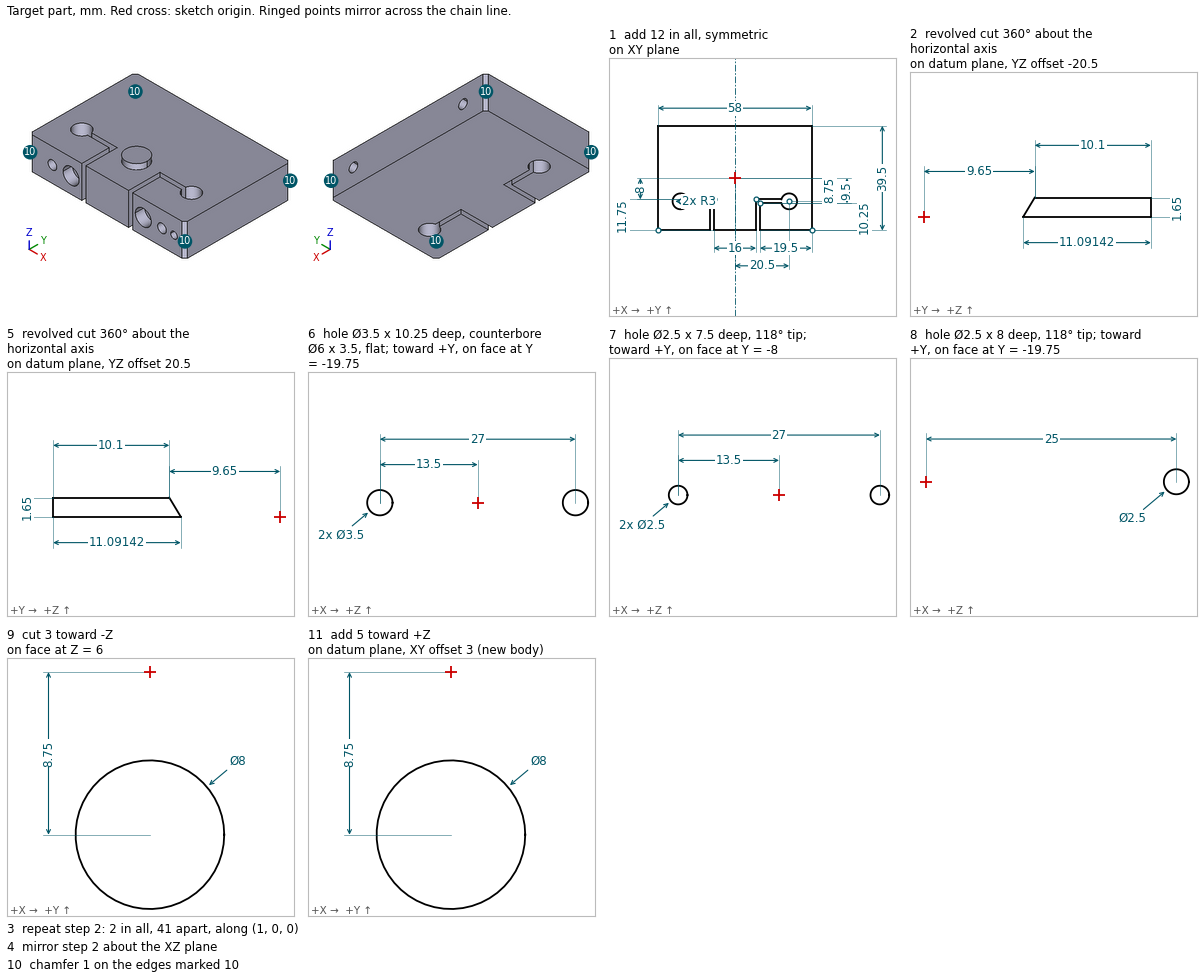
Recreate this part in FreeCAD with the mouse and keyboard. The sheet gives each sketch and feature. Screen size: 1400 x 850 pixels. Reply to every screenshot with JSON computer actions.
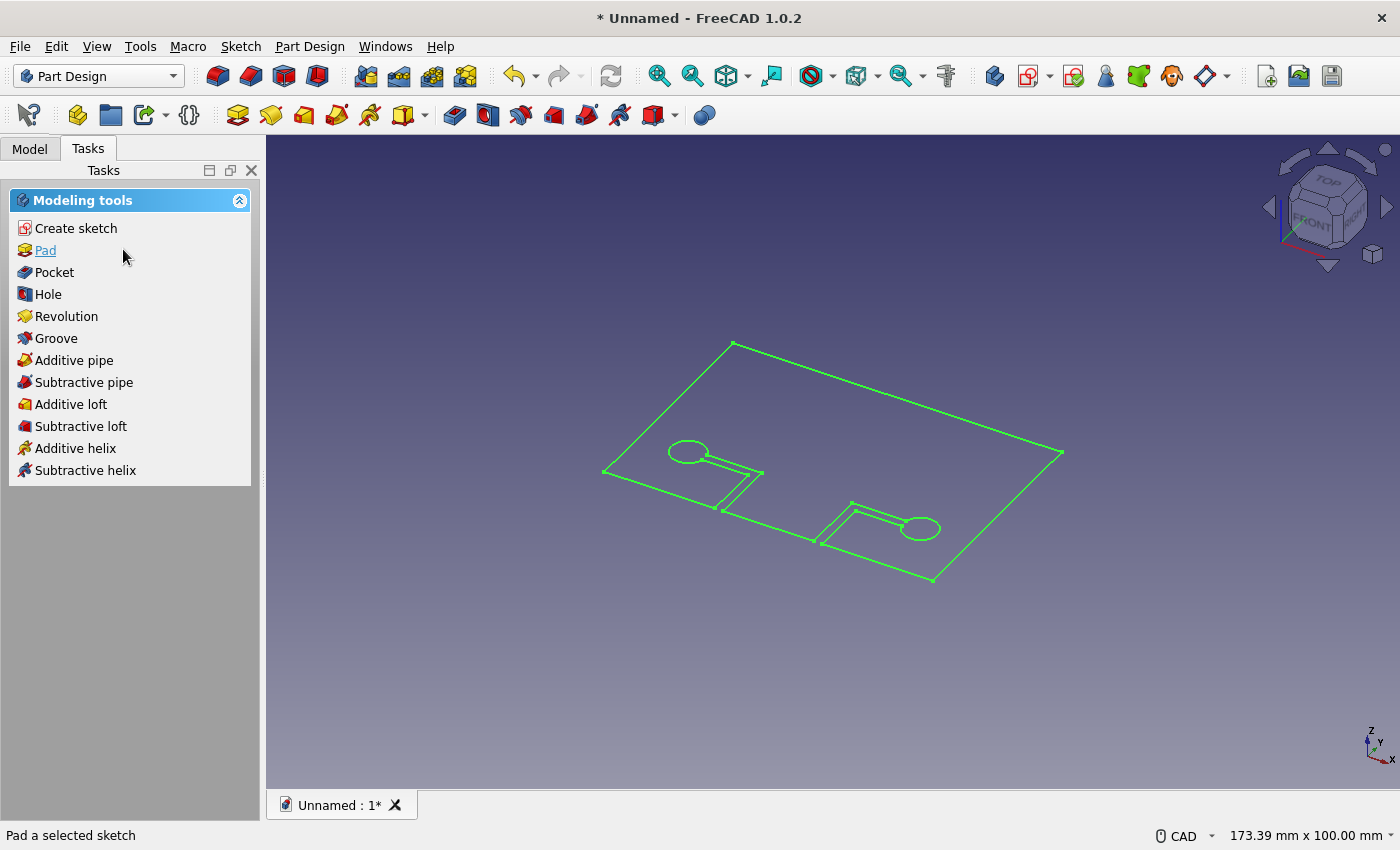
{"action": "left_click", "coordinate": [238, 116]}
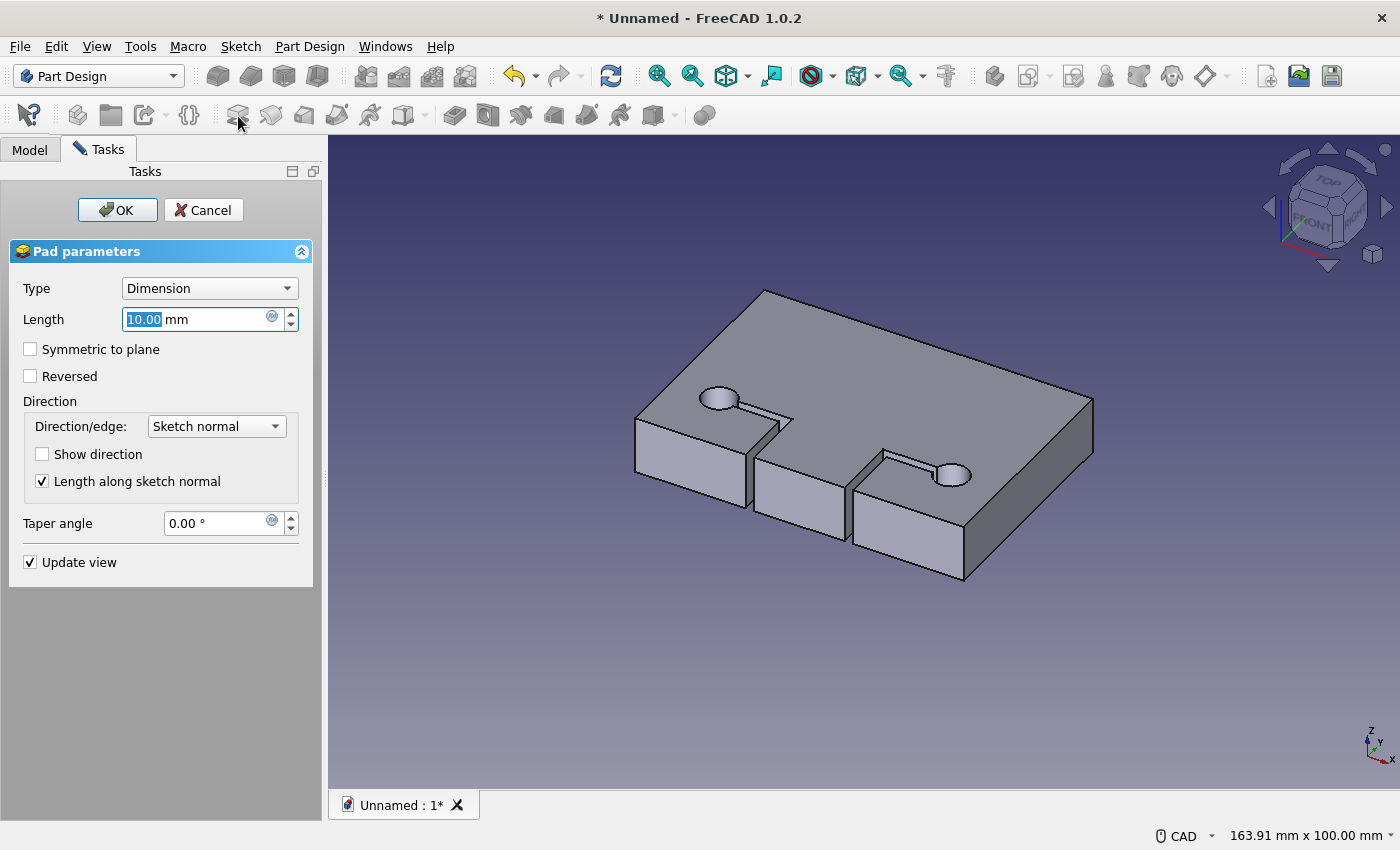
{"action": "type", "text": "12"}
{"action": "key", "text": "Tab"}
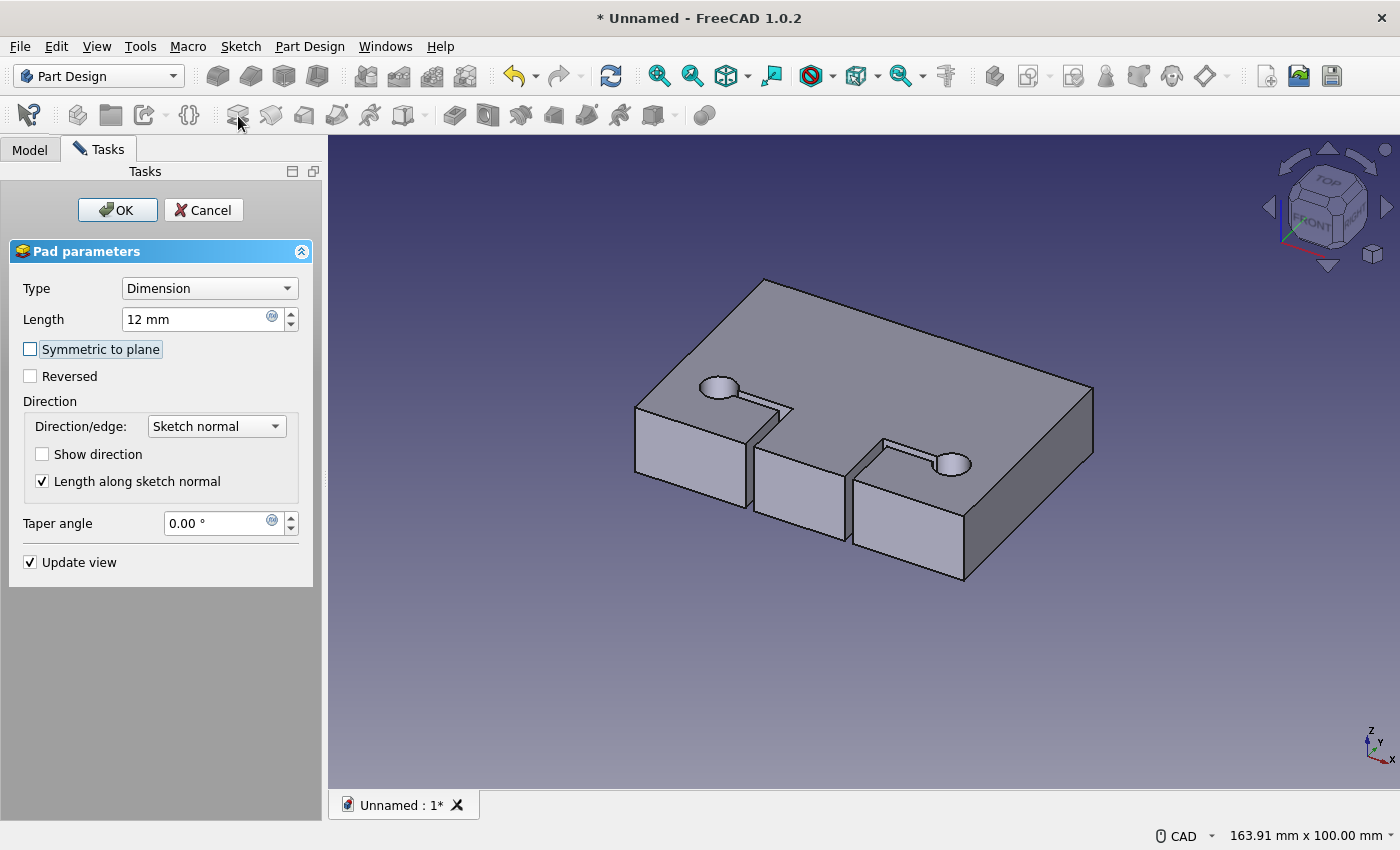
{"action": "left_click", "coordinate": [31, 349]}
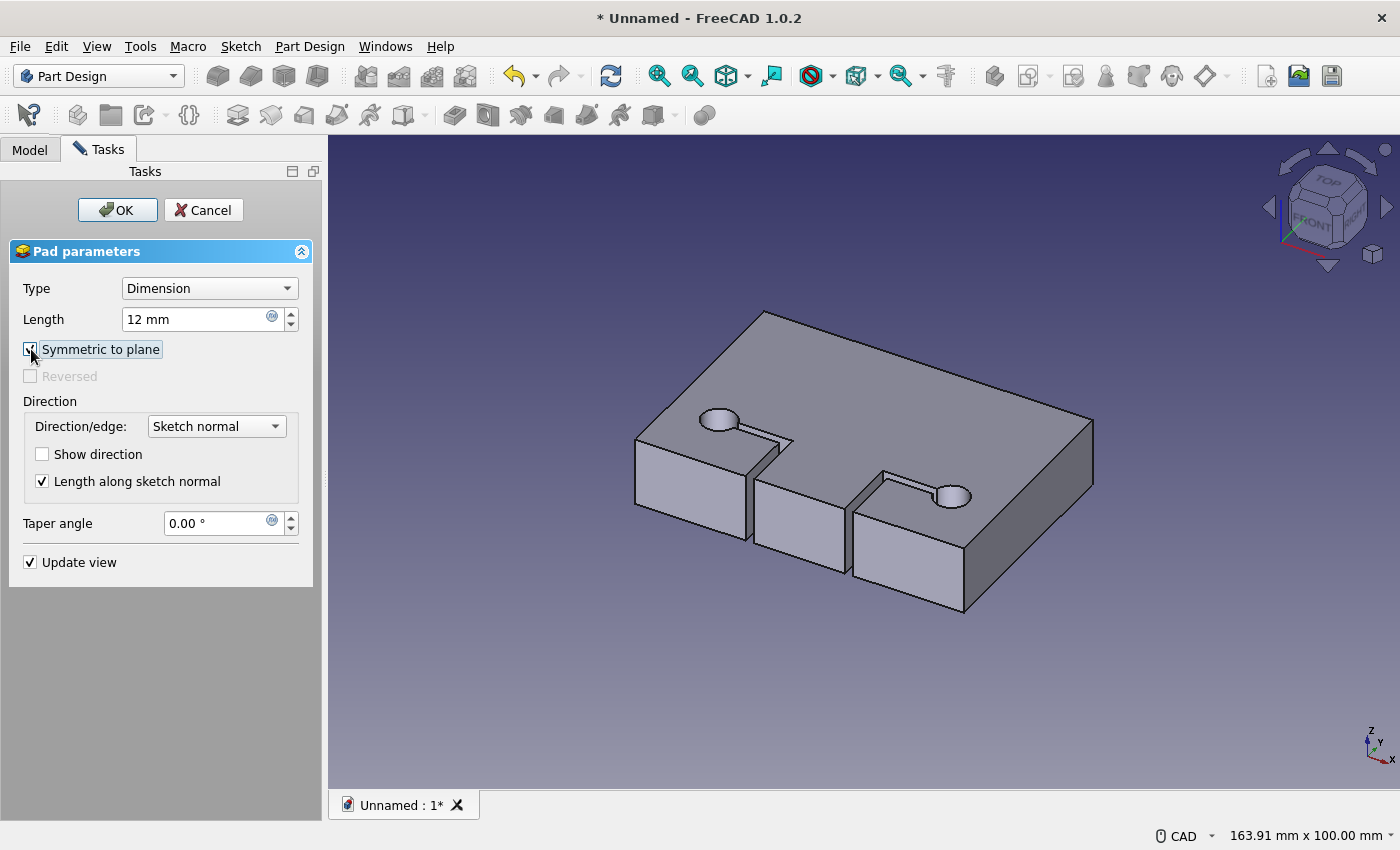
{"action": "left_click", "coordinate": [118, 210]}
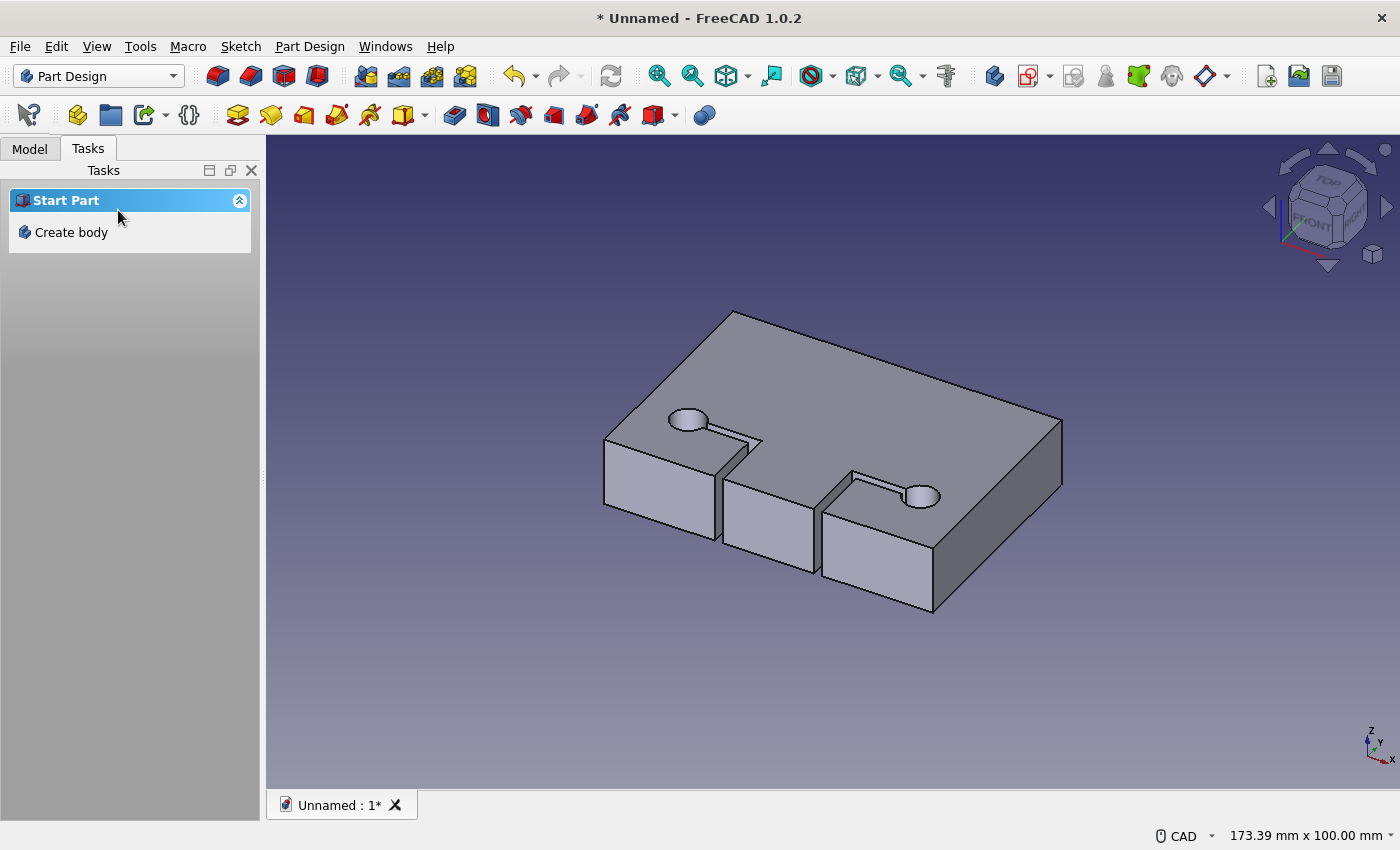
{"action": "left_click", "coordinate": [30, 148]}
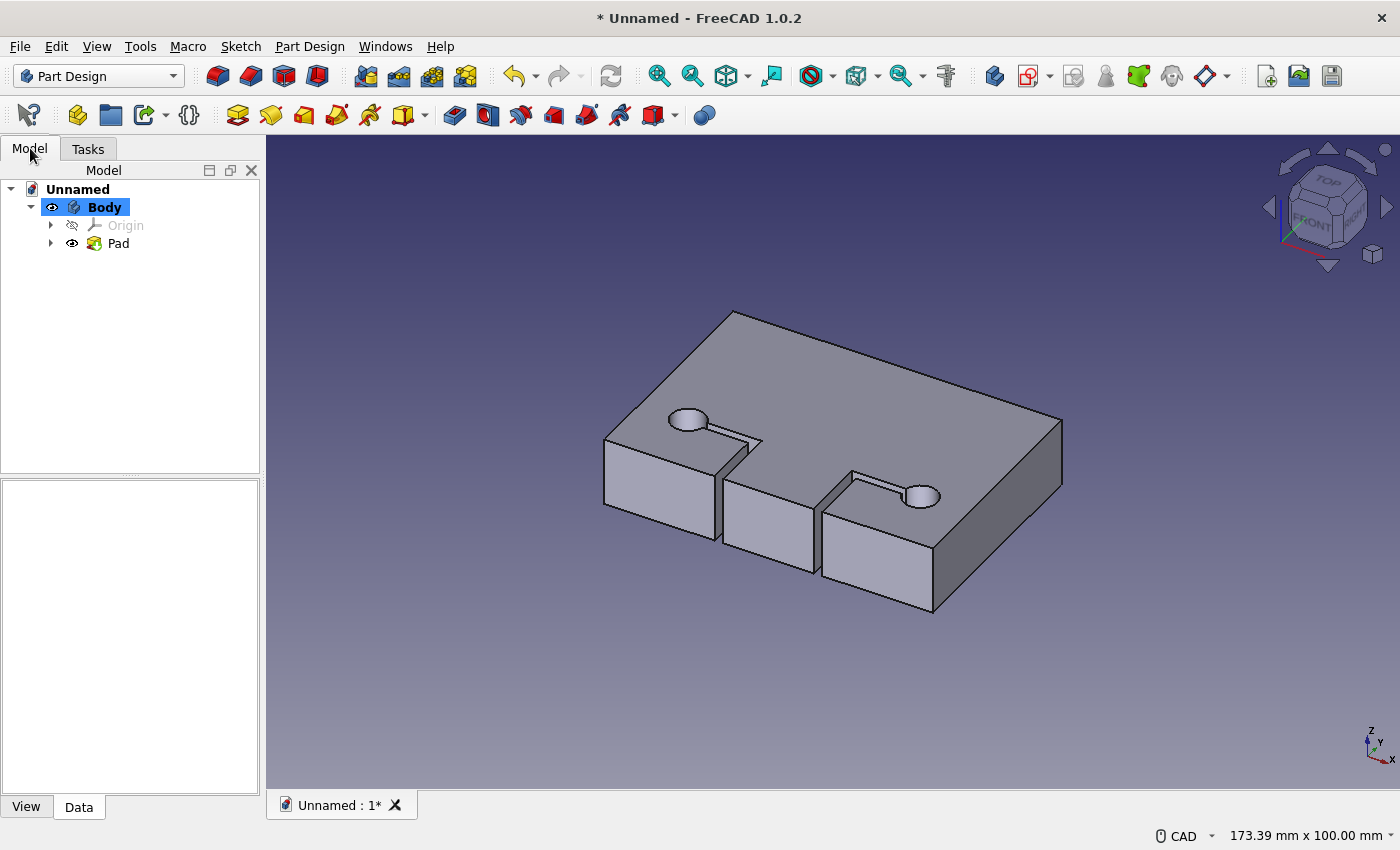
{"action": "left_click", "coordinate": [51, 225]}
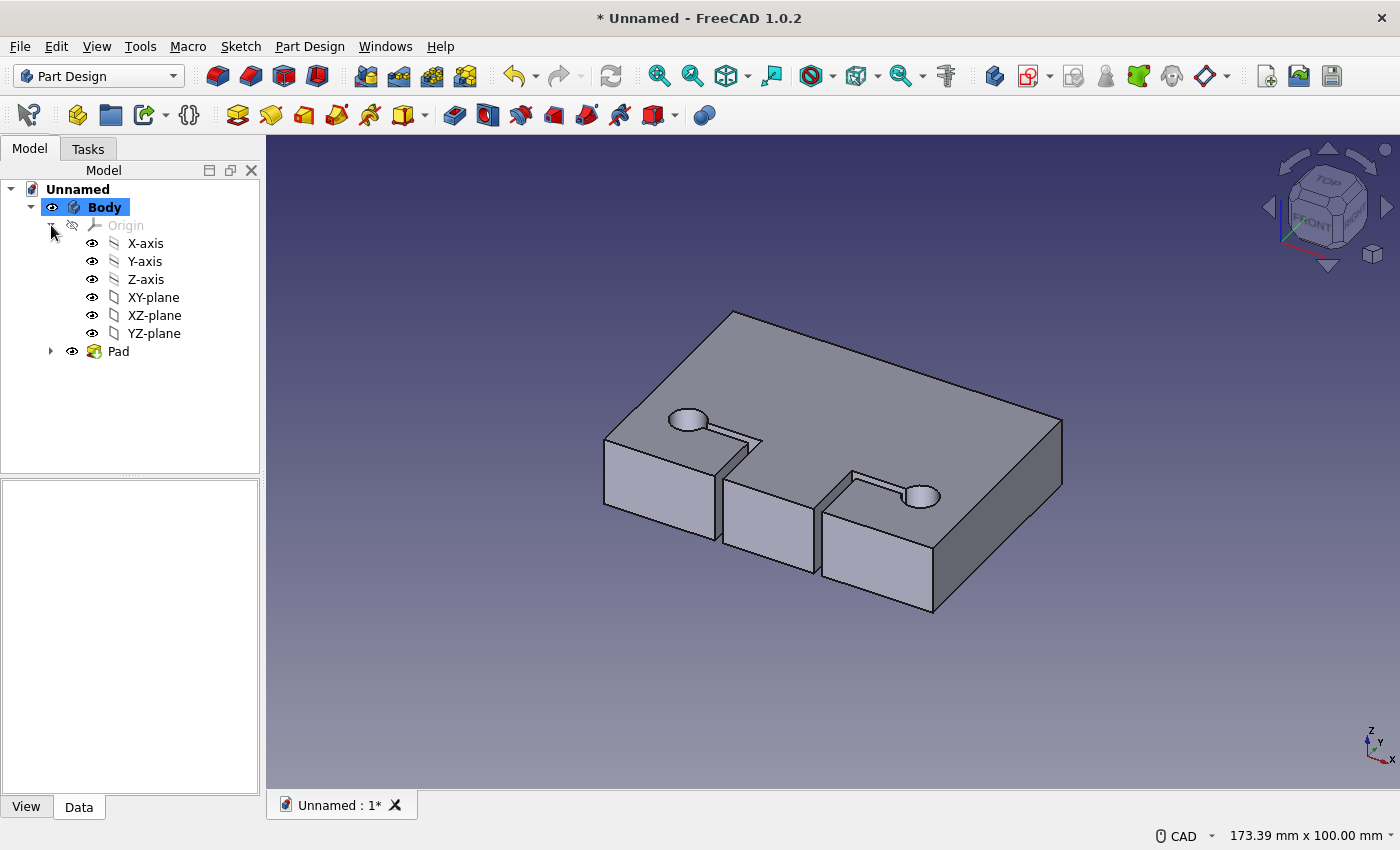
{"action": "left_click", "coordinate": [137, 333]}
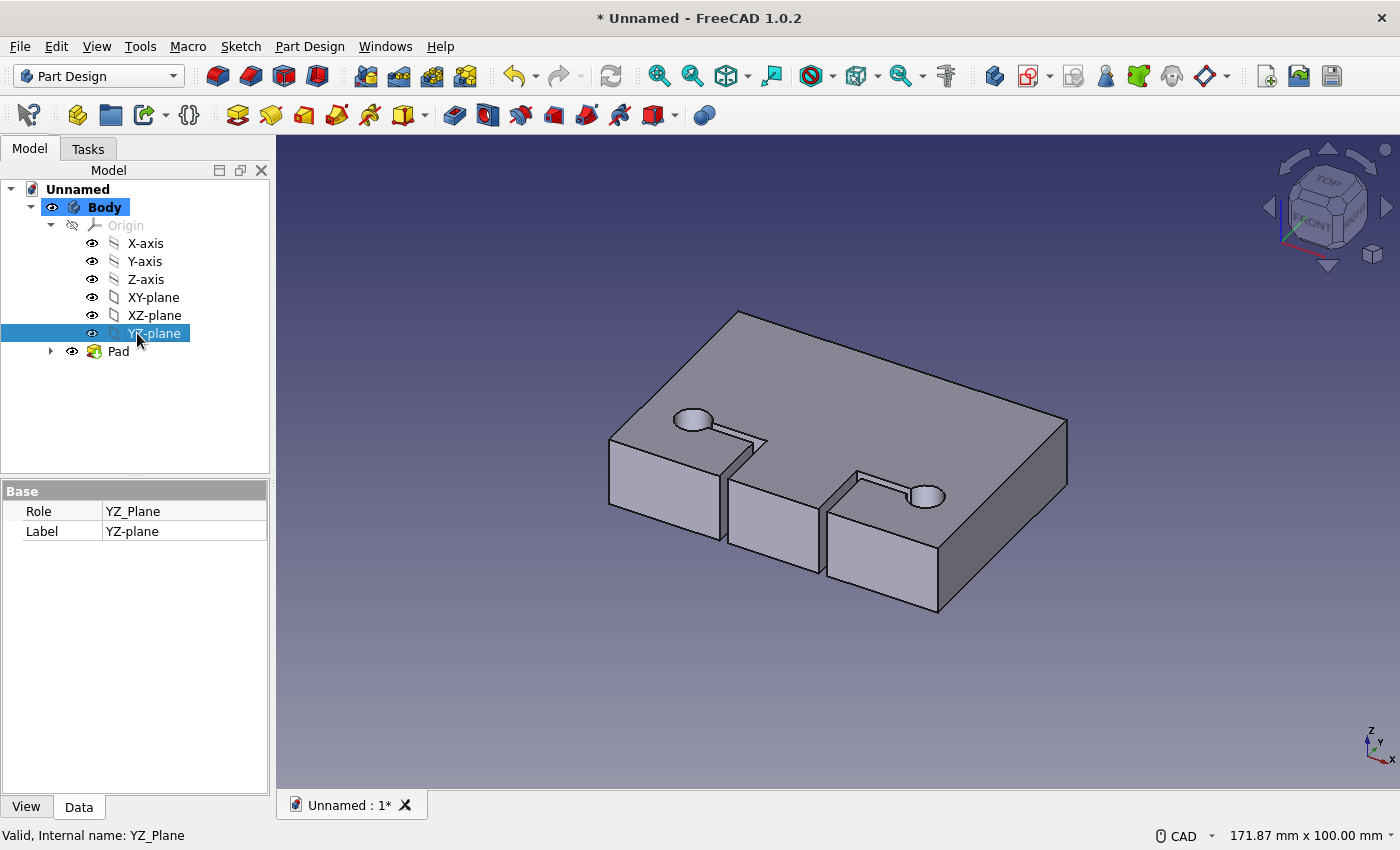
{"action": "left_click", "coordinate": [1204, 76]}